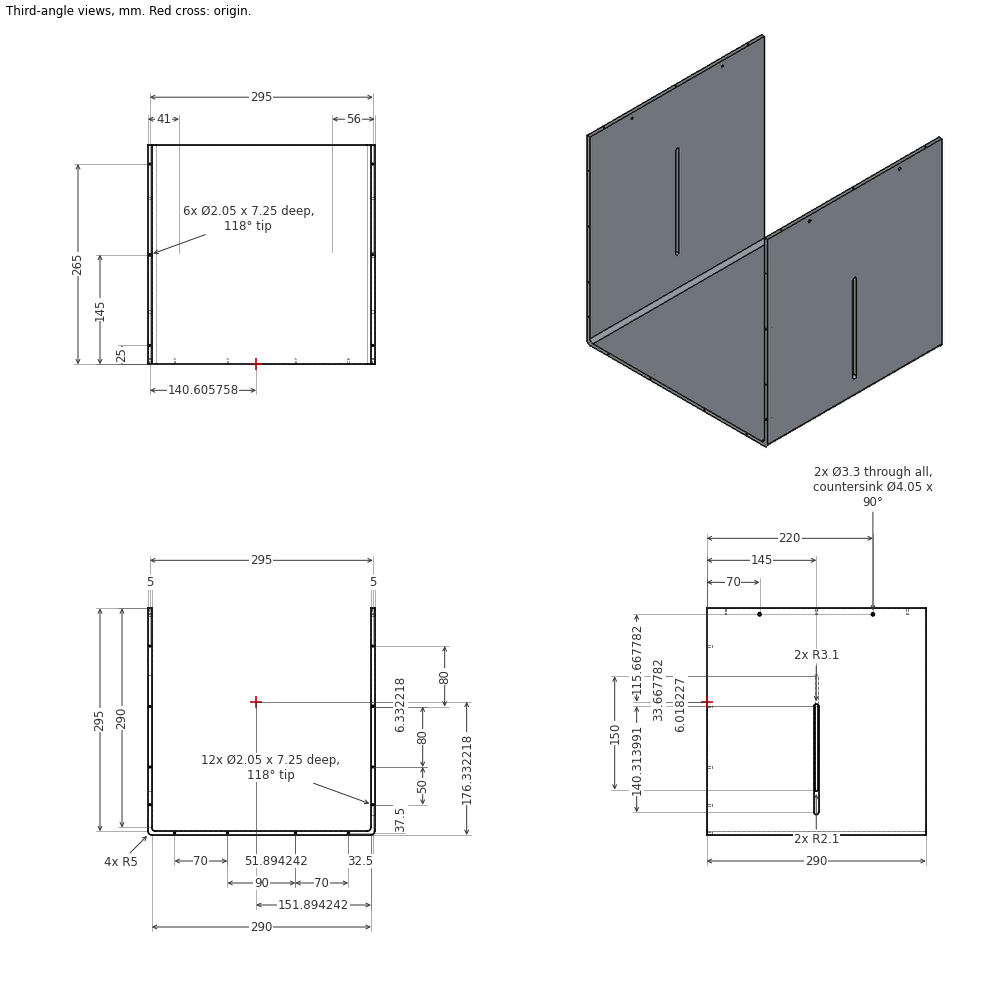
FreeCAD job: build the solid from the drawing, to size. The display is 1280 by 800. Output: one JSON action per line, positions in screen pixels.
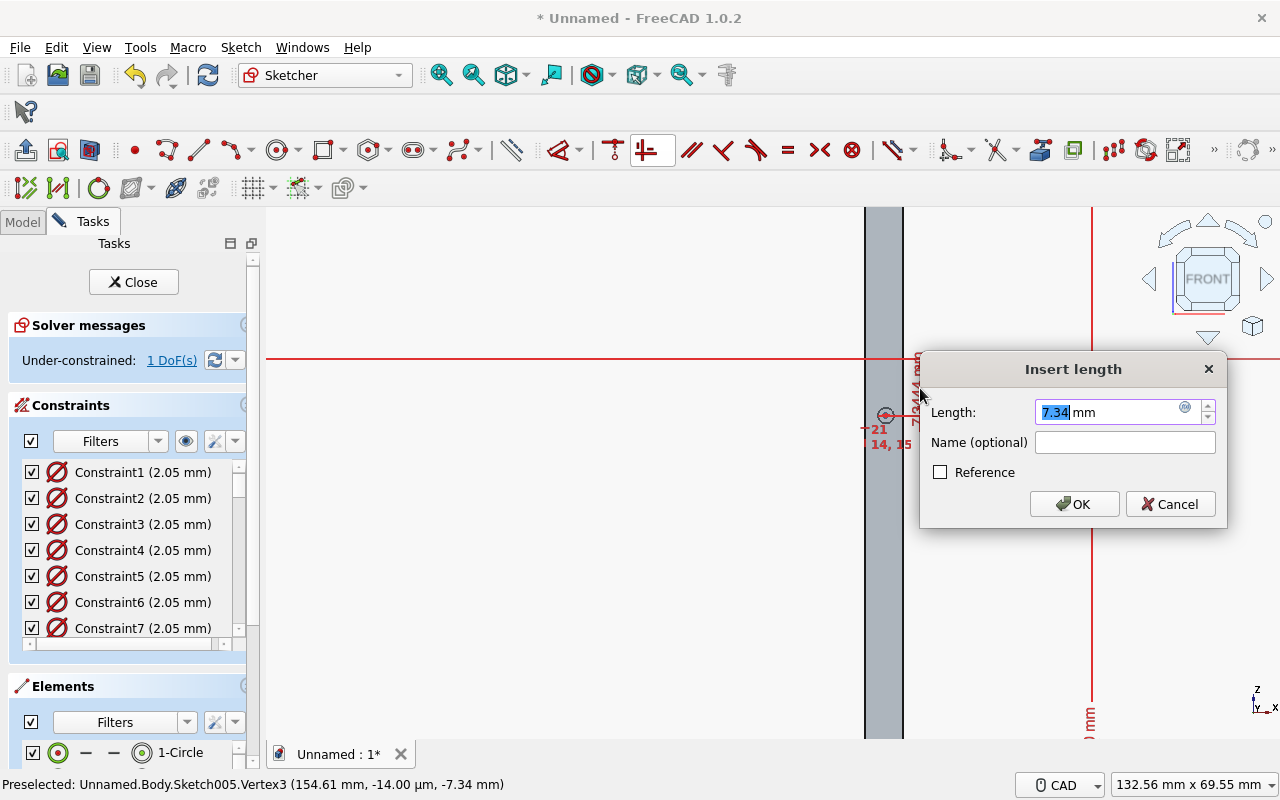
{"action": "type", "text": "6.332218"}
{"action": "key", "text": "Return"}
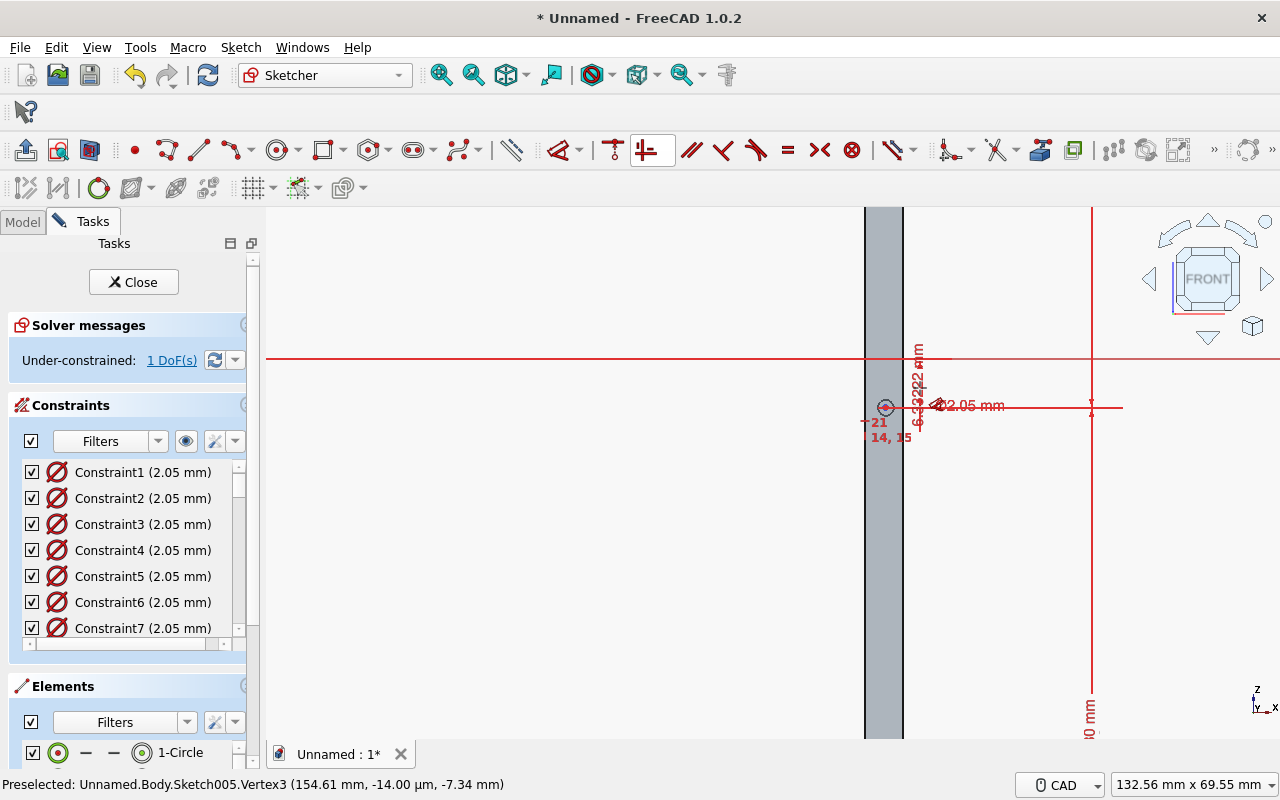
{"action": "scroll", "coordinate": [892, 420], "scroll_direction": "down", "scroll_amount": 9}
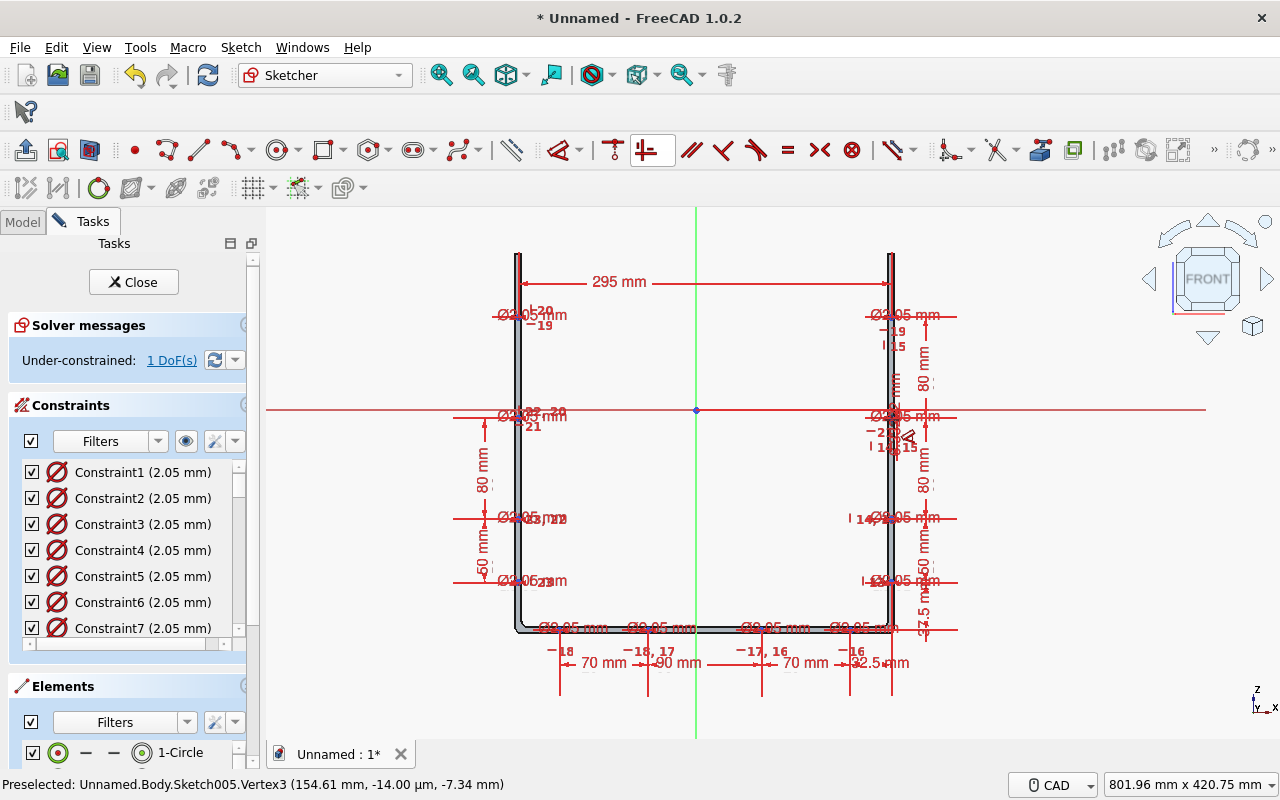
{"action": "left_click", "coordinate": [762, 630]}
{"action": "left_click", "coordinate": [729, 376]}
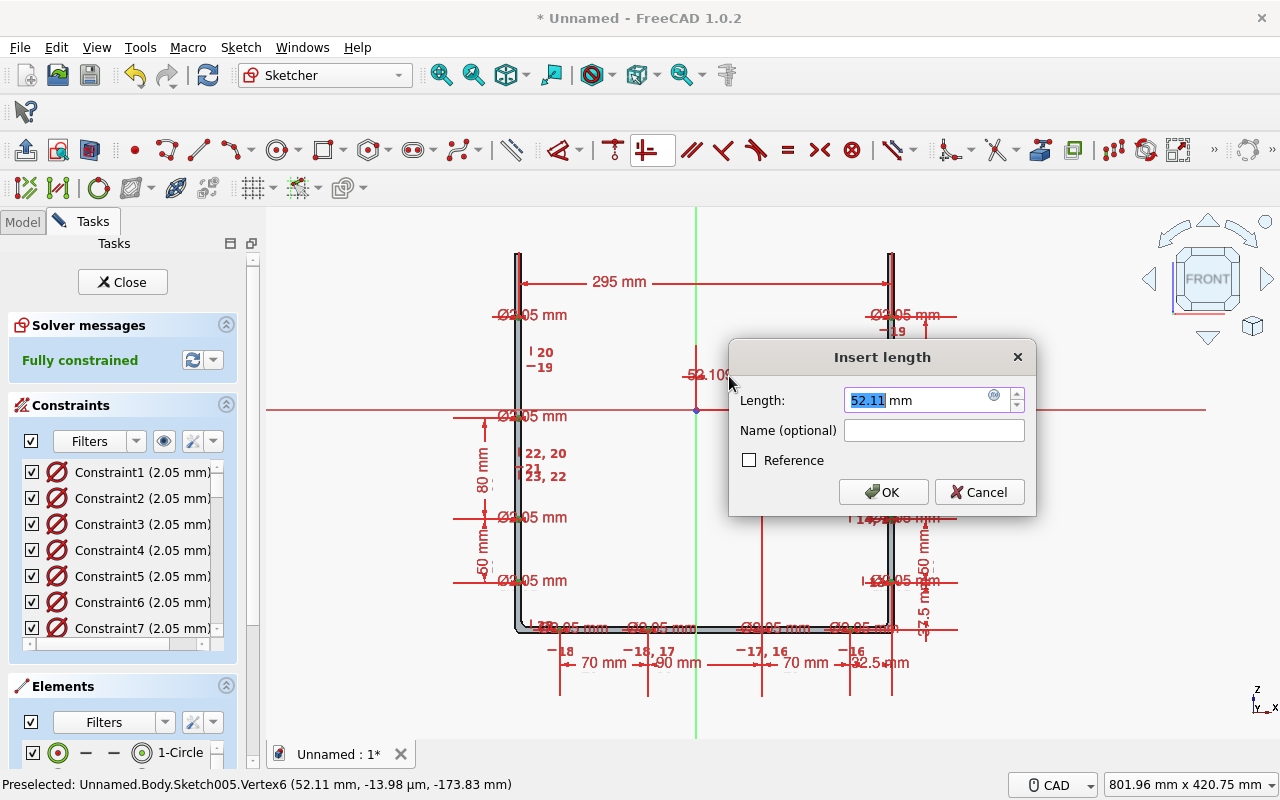
{"action": "type", "text": "51.894242"}
{"action": "key", "text": "Return"}
{"action": "key", "text": "Escape"}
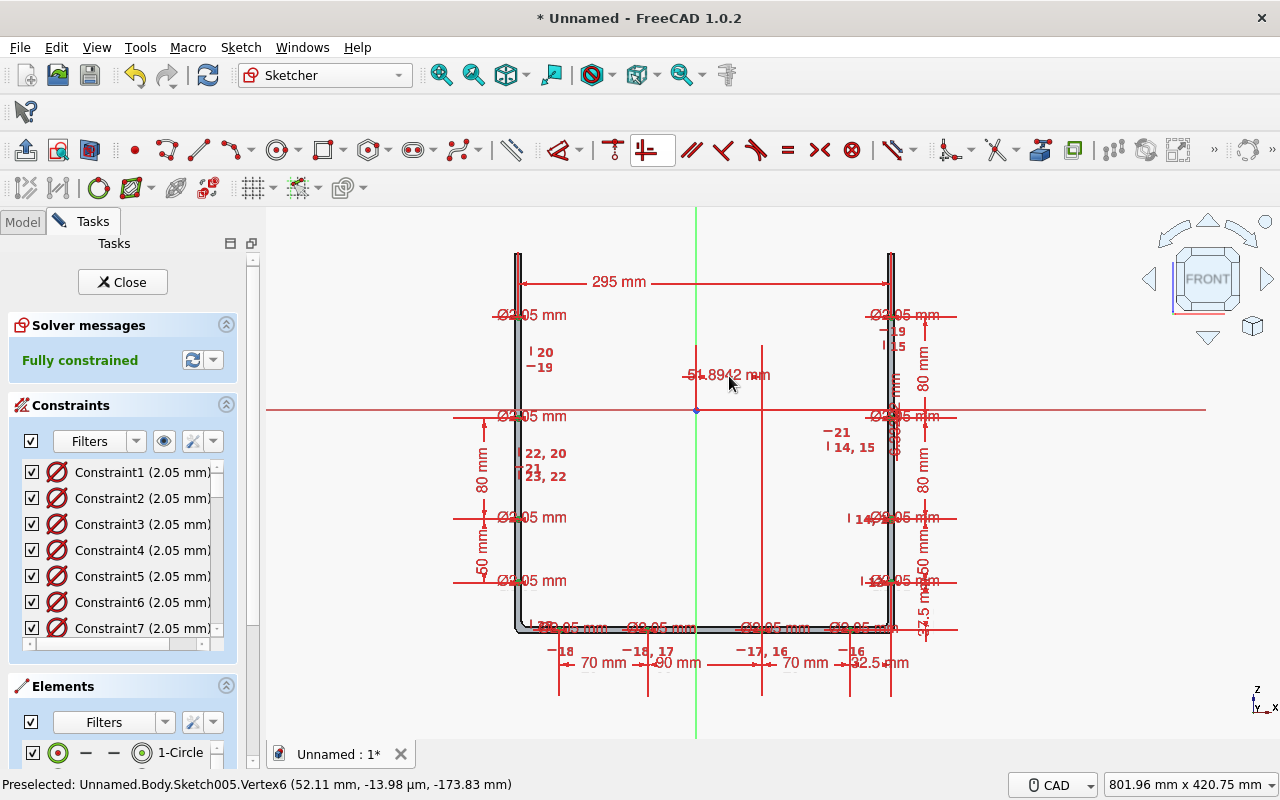
{"action": "left_click", "coordinate": [123, 282]}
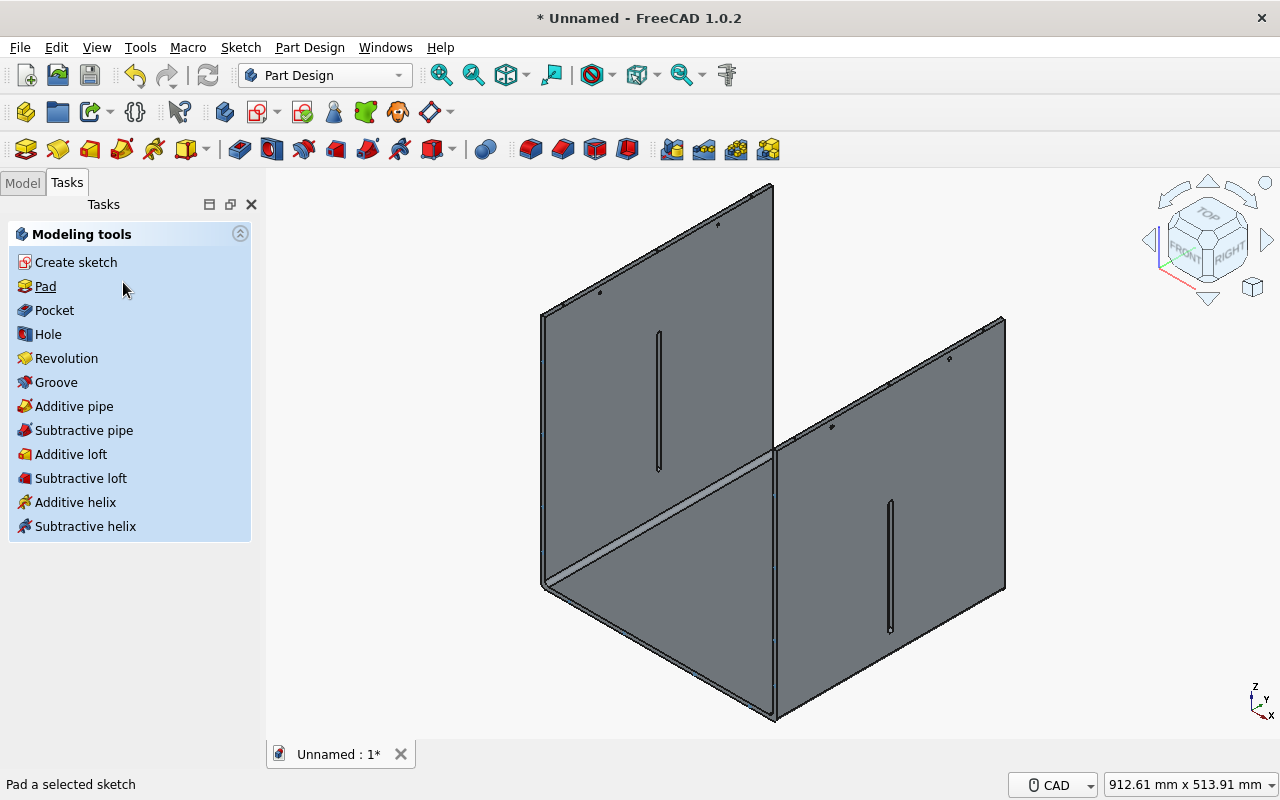
{"action": "left_click", "coordinate": [272, 150]}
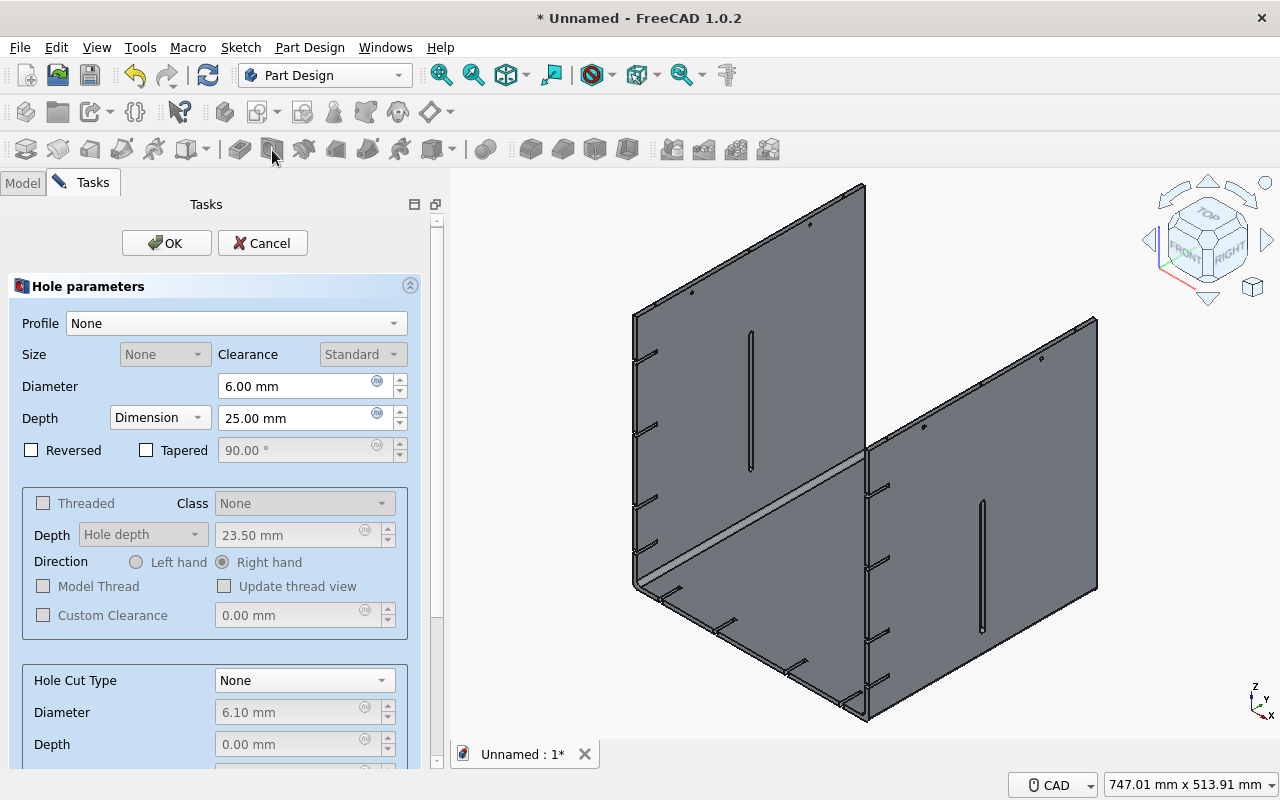
{"action": "triple_click", "coordinate": [305, 386]}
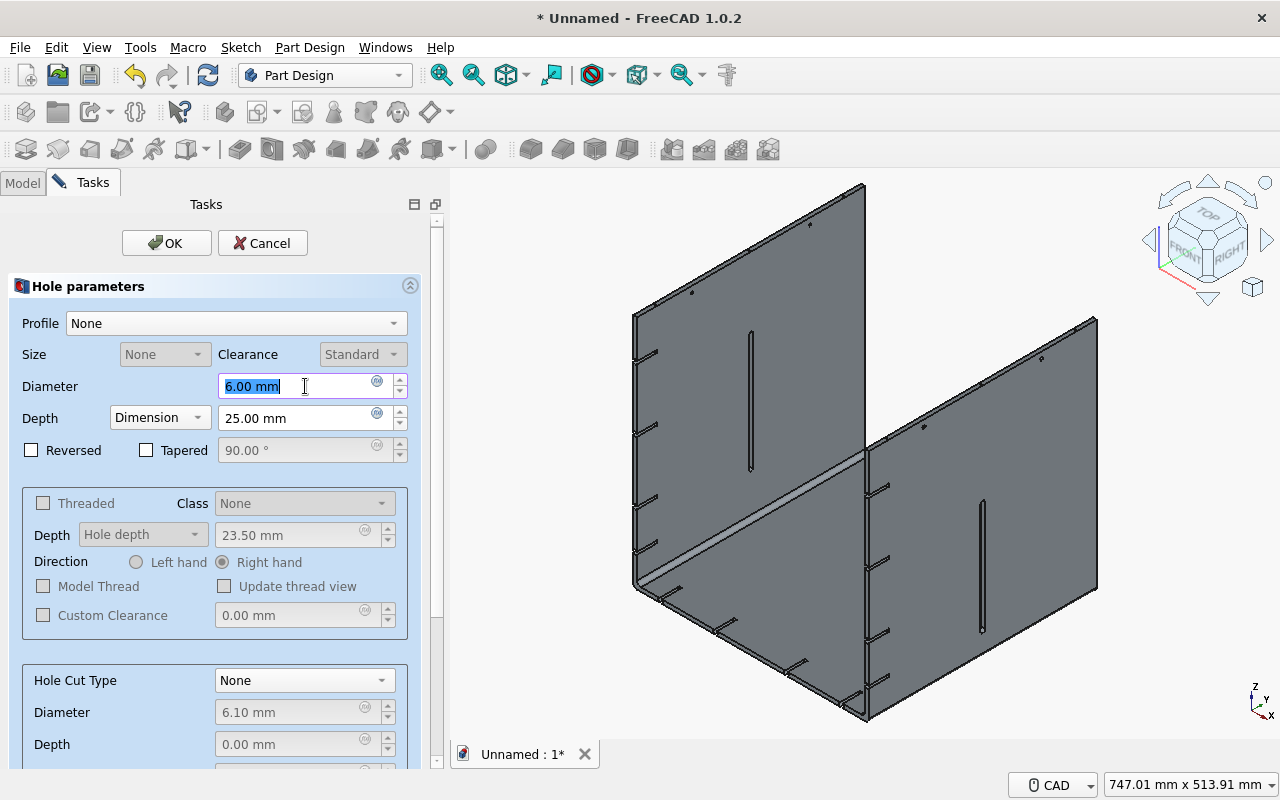
{"action": "type", "text": "2.05"}
{"action": "key", "text": "Tab"}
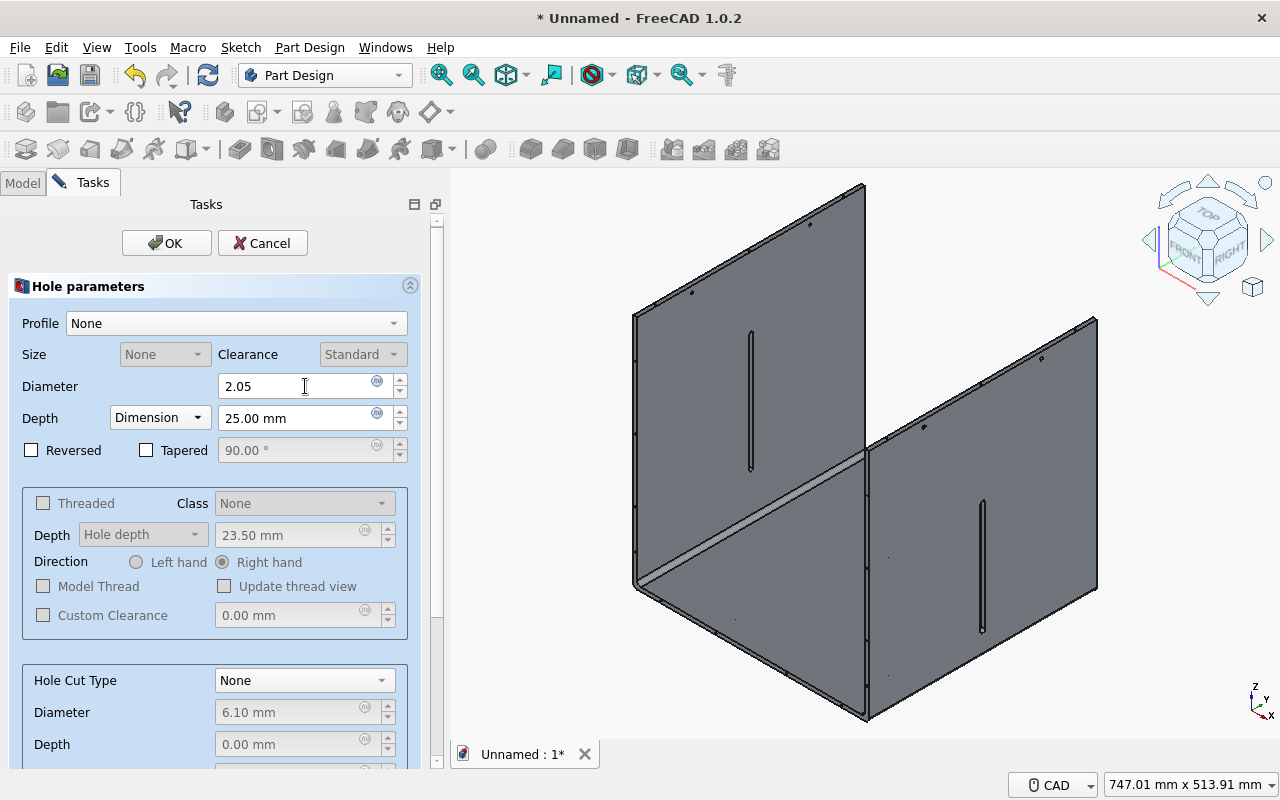
{"action": "triple_click", "coordinate": [305, 418]}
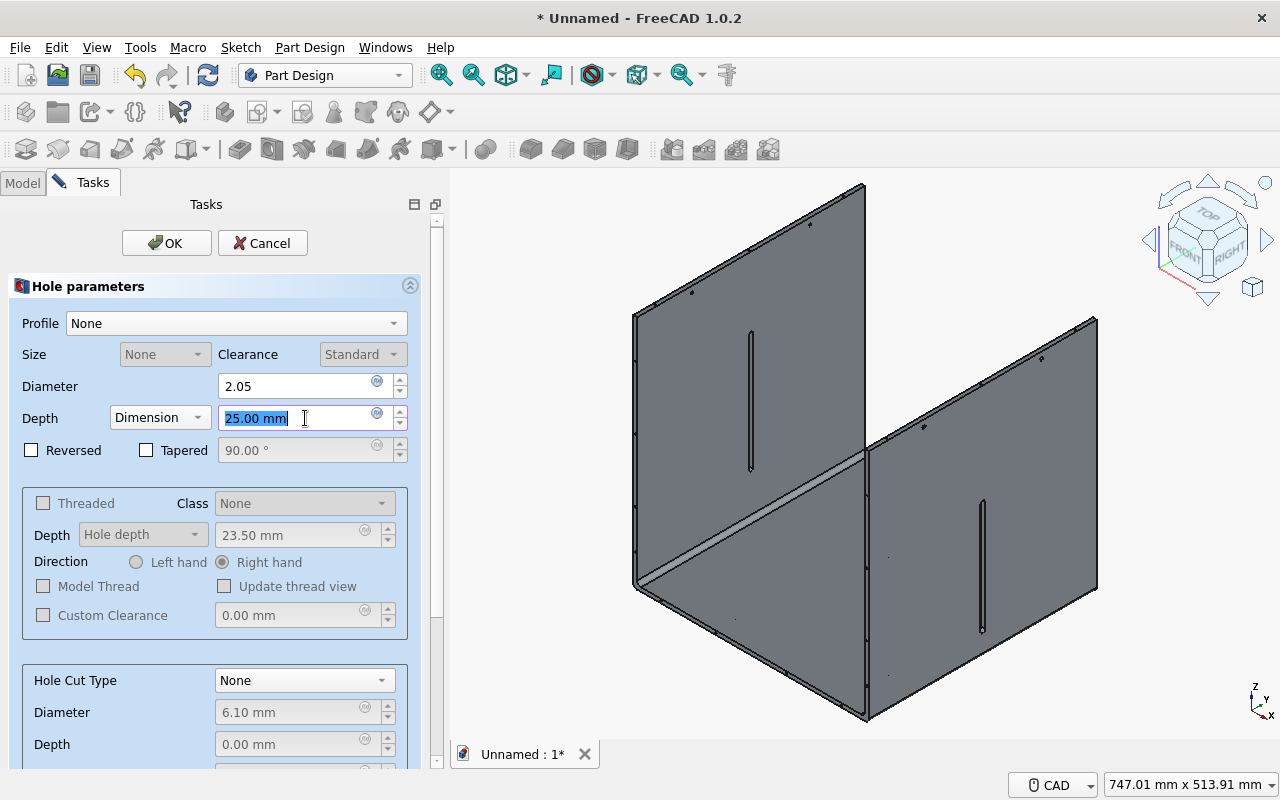
{"action": "type", "text": "7.25"}
{"action": "key", "text": "Tab"}